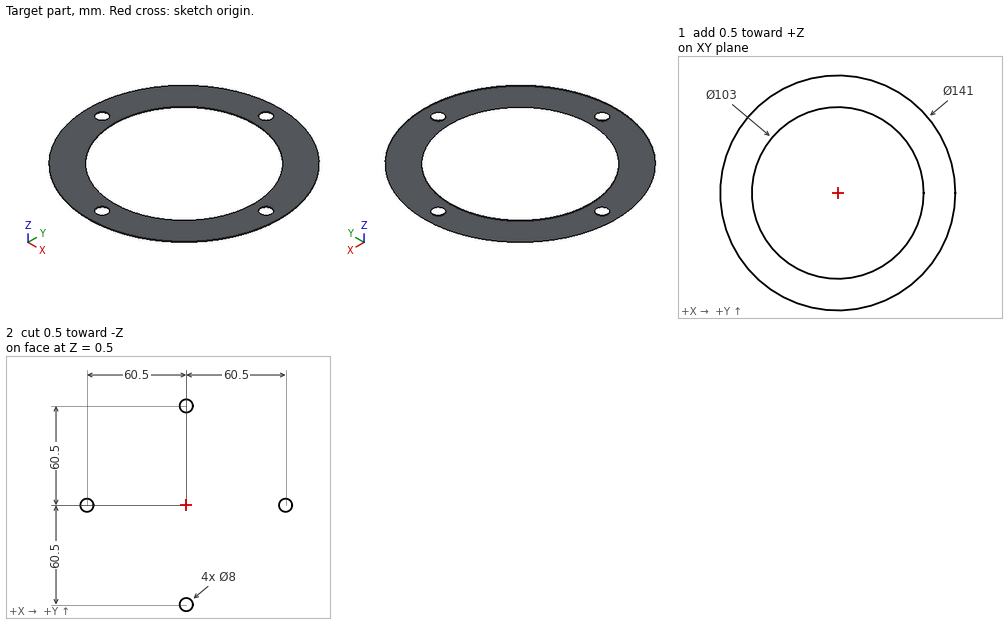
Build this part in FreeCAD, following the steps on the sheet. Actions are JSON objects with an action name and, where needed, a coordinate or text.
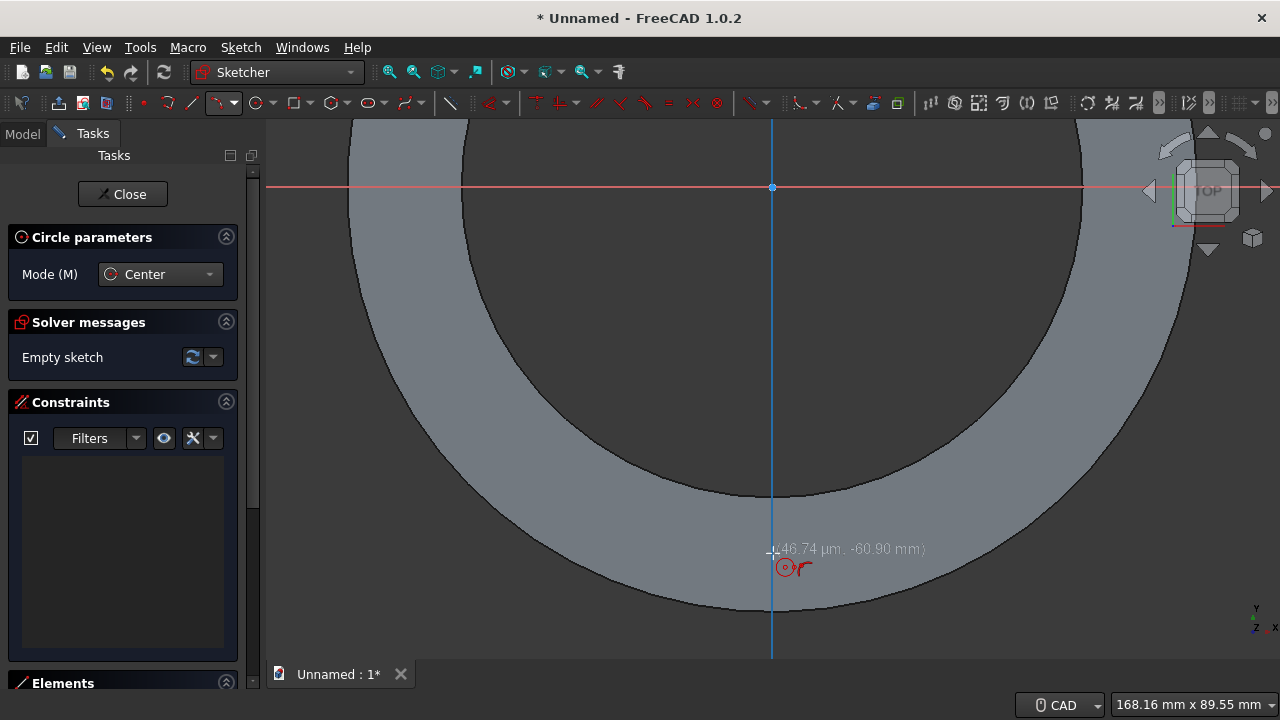
{"action": "left_click", "coordinate": [772, 552]}
{"action": "left_click", "coordinate": [789, 535]}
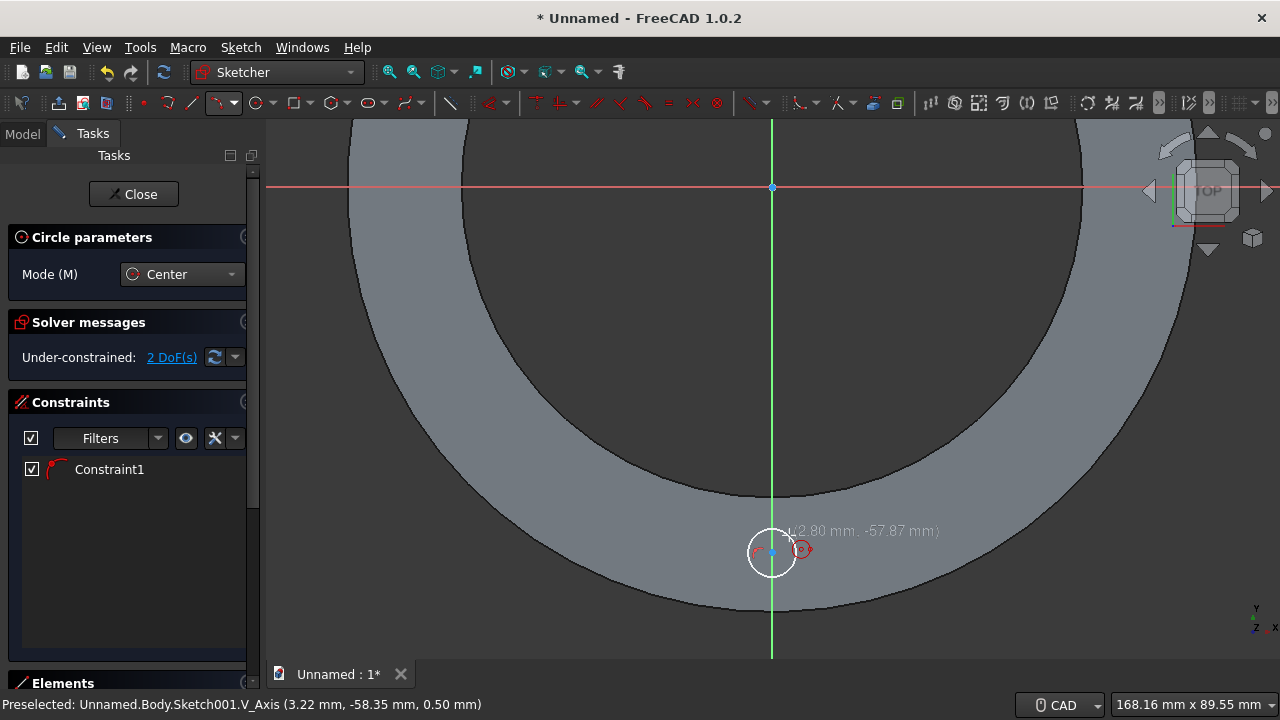
{"action": "left_click", "coordinate": [407, 187]}
{"action": "left_click", "coordinate": [424, 170]}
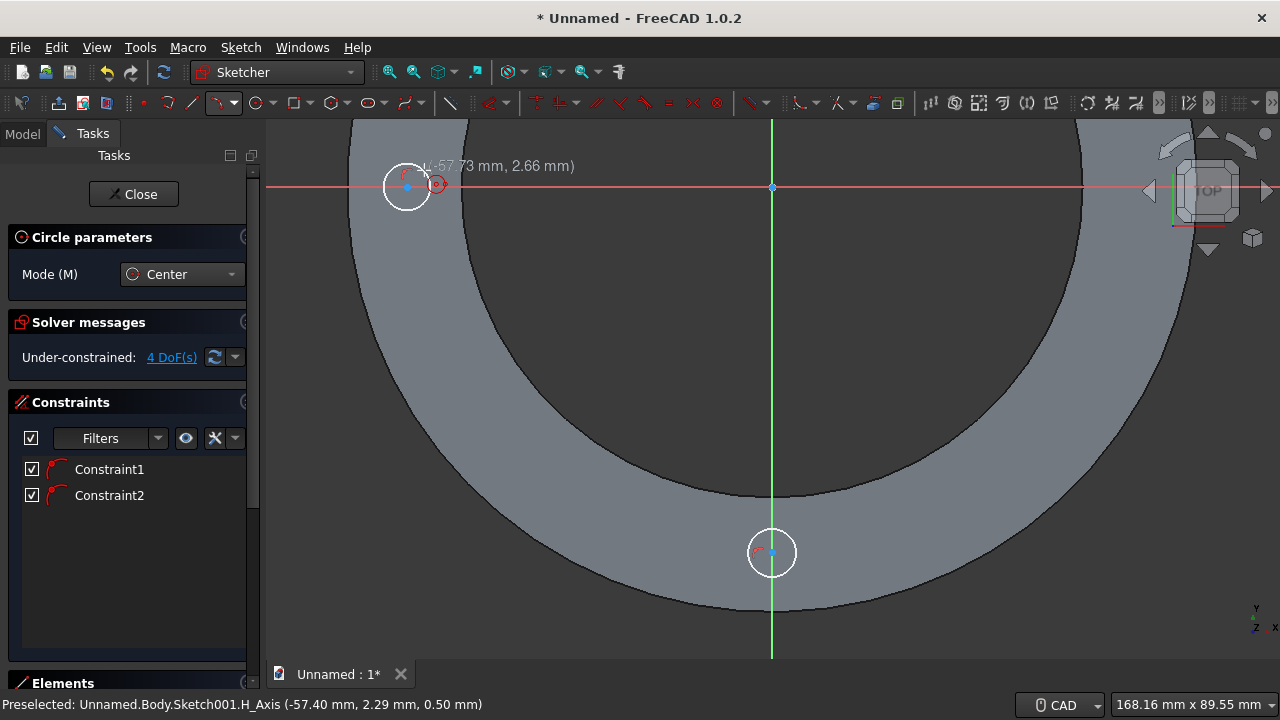
{"action": "scroll", "coordinate": [649, 554], "scroll_direction": "down", "scroll_amount": 4}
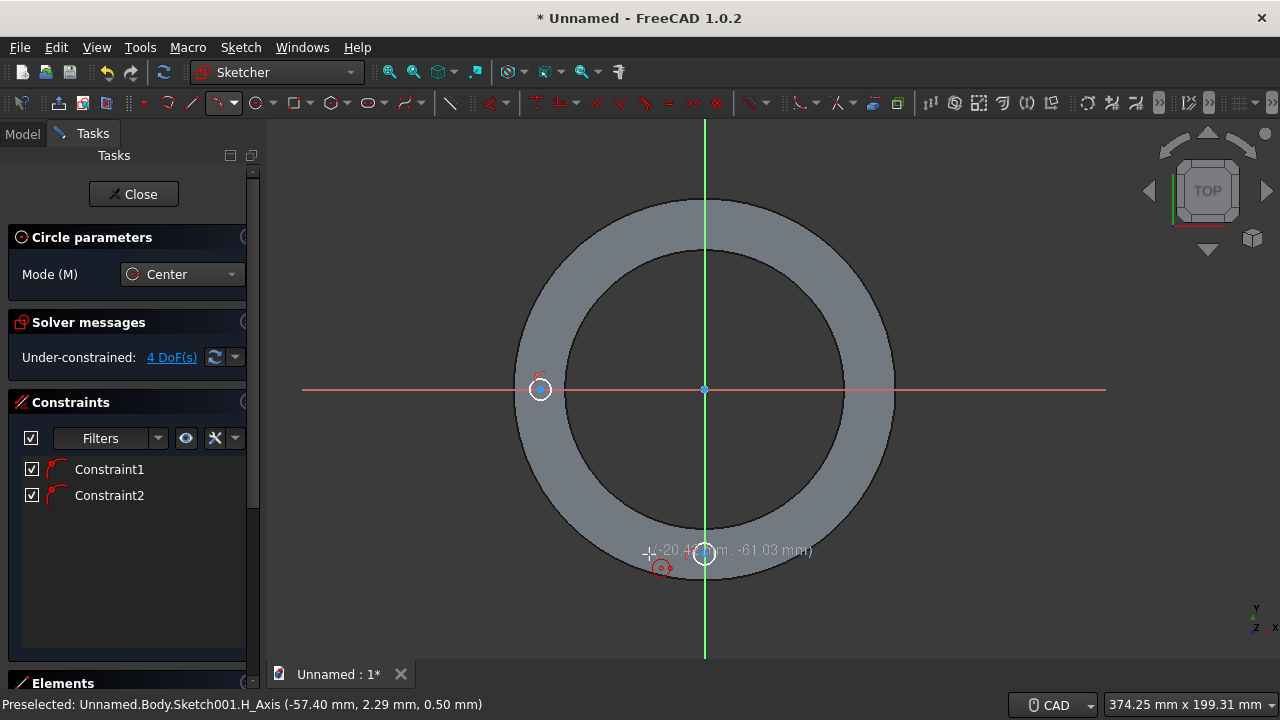
{"action": "scroll", "coordinate": [705, 226], "scroll_direction": "up", "scroll_amount": 4}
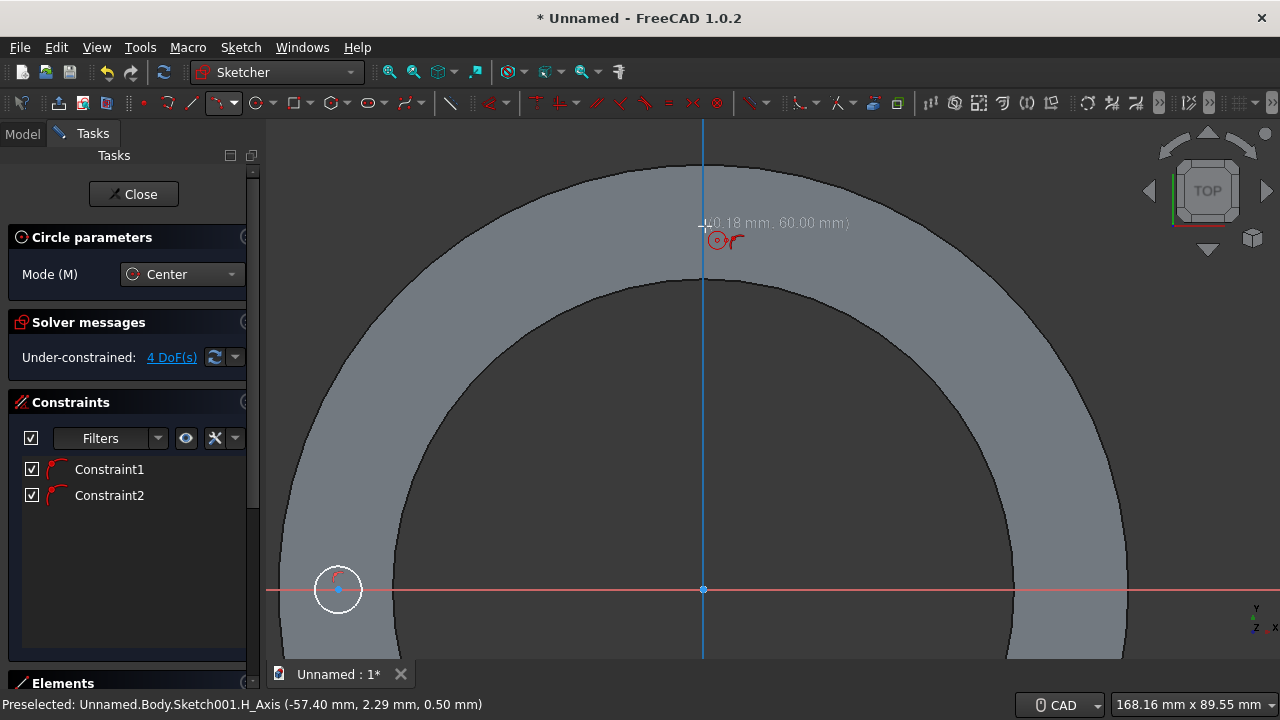
{"action": "left_click", "coordinate": [703, 225]}
{"action": "left_click", "coordinate": [720, 208]}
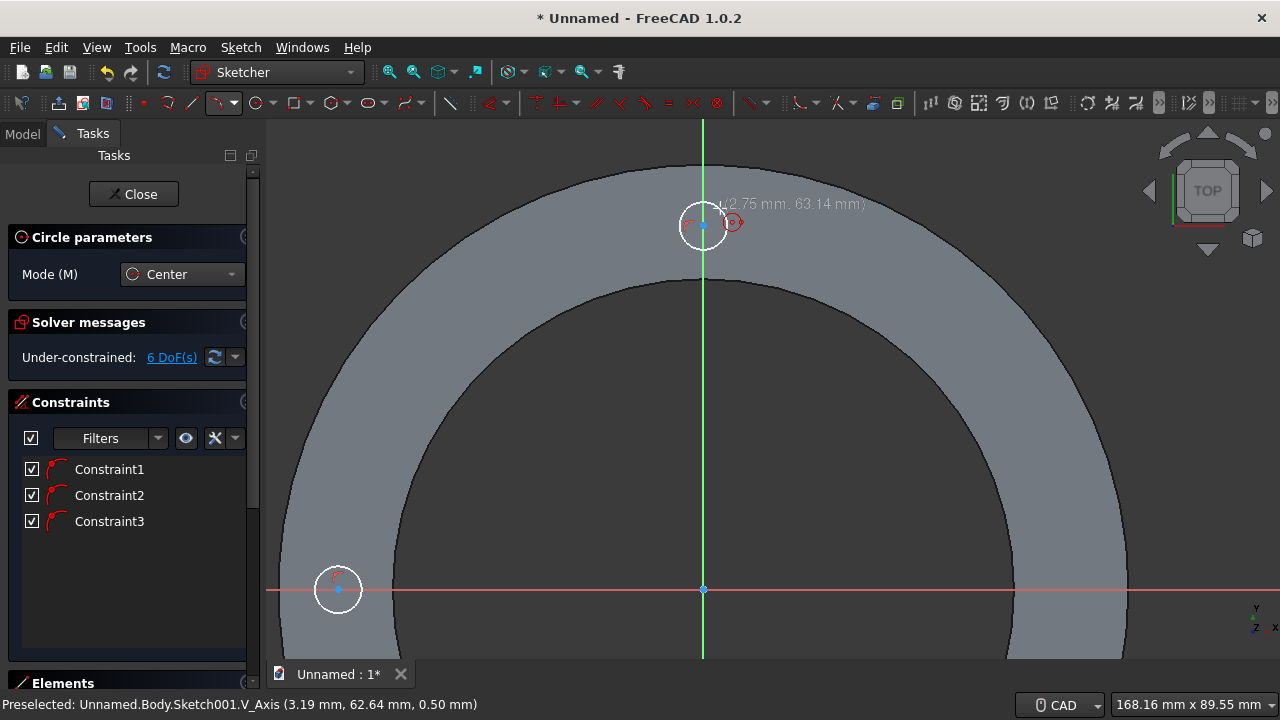
{"action": "left_click", "coordinate": [1068, 590]}
{"action": "left_click", "coordinate": [1085, 573]}
{"action": "key", "text": "Escape"}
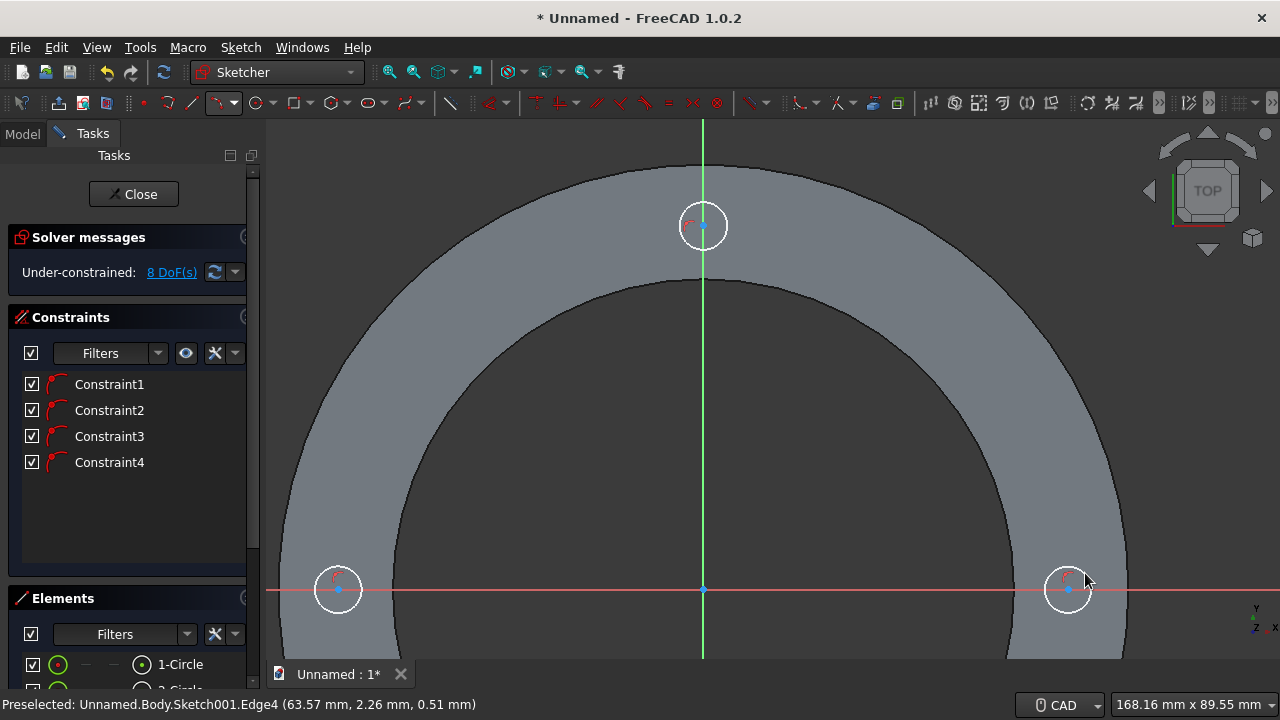
{"action": "scroll", "coordinate": [705, 225], "scroll_direction": "down", "scroll_amount": 4}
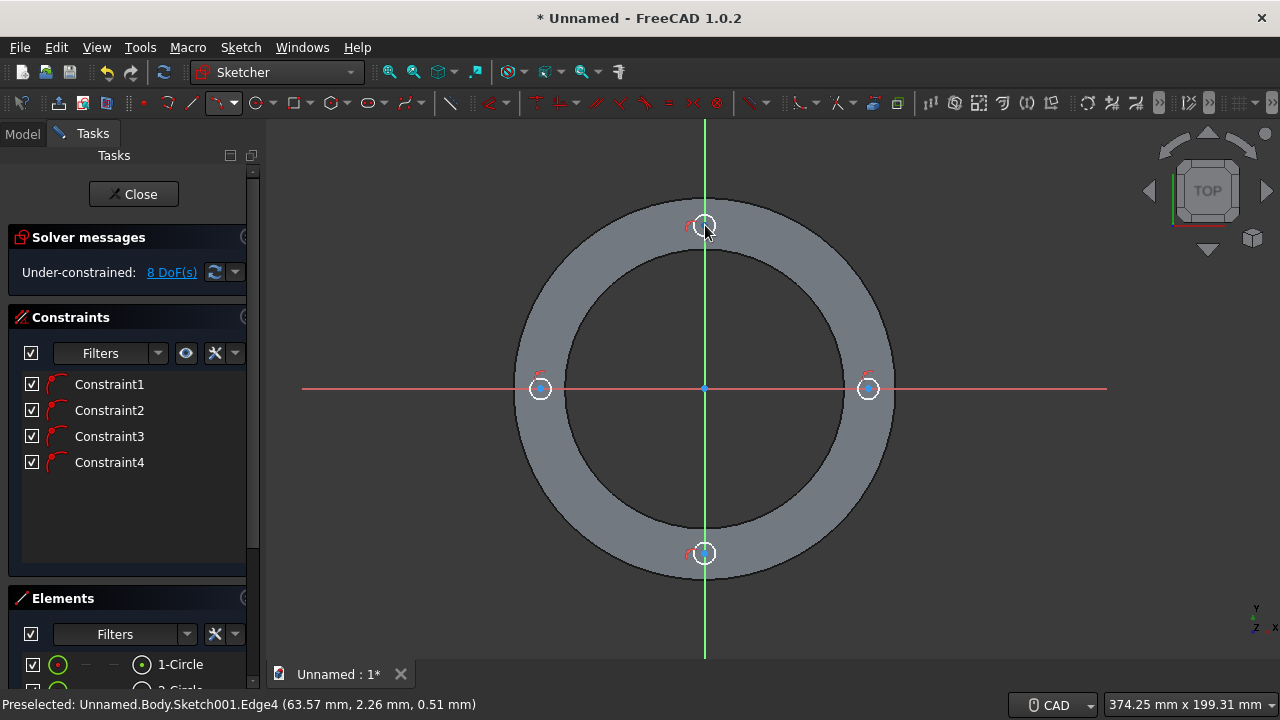
{"action": "scroll", "coordinate": [712, 546], "scroll_direction": "up", "scroll_amount": 3}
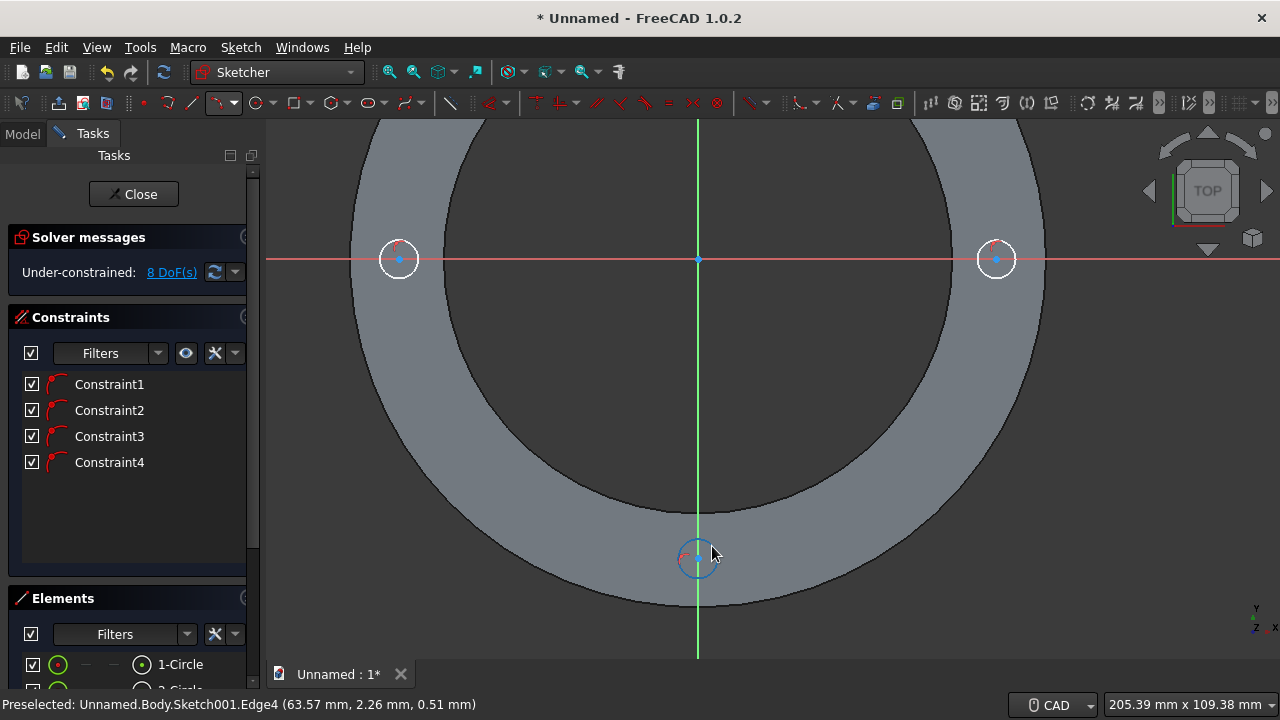
{"action": "left_click", "coordinate": [712, 545]}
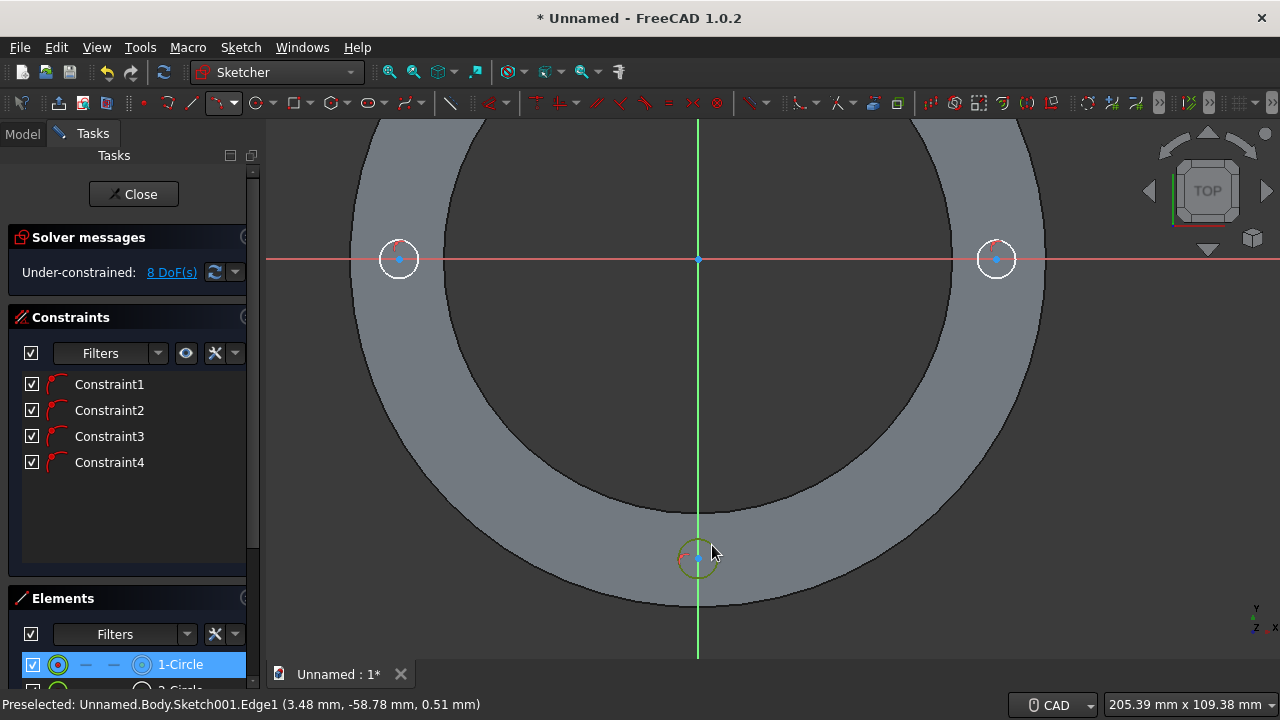
{"action": "left_click", "coordinate": [413, 246]}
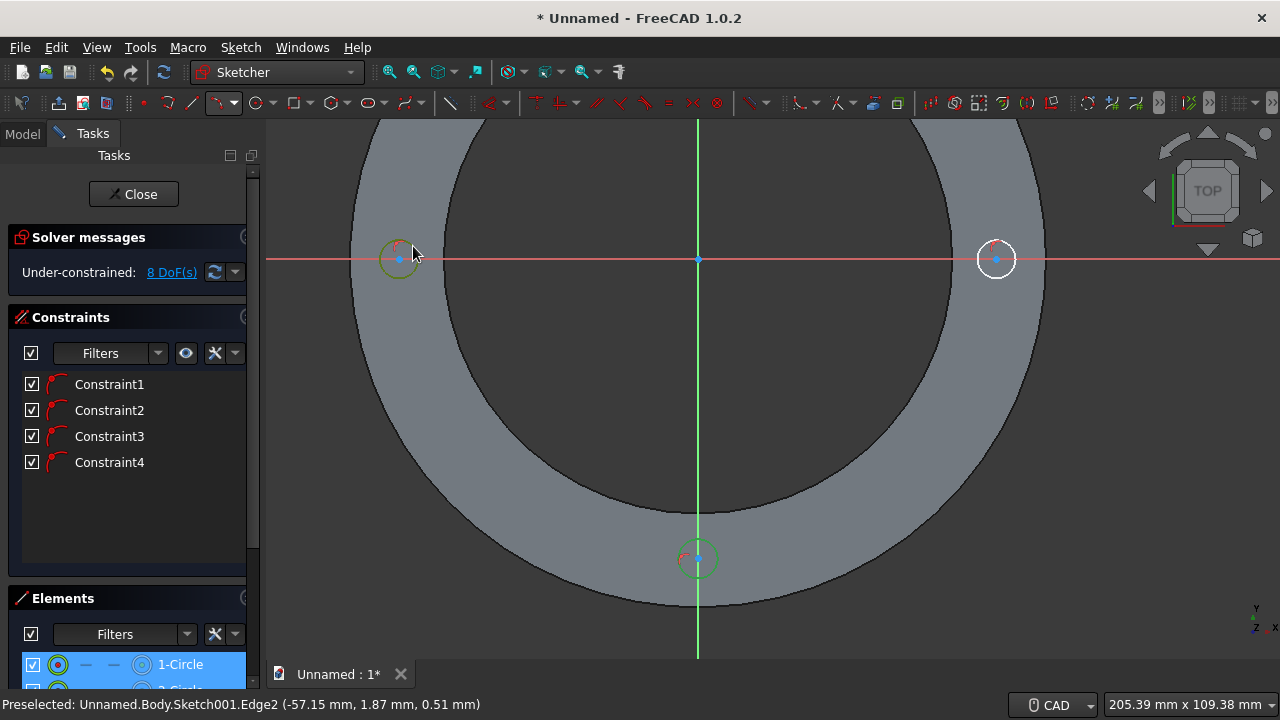
{"action": "scroll", "coordinate": [712, 547], "scroll_direction": "down", "scroll_amount": 3}